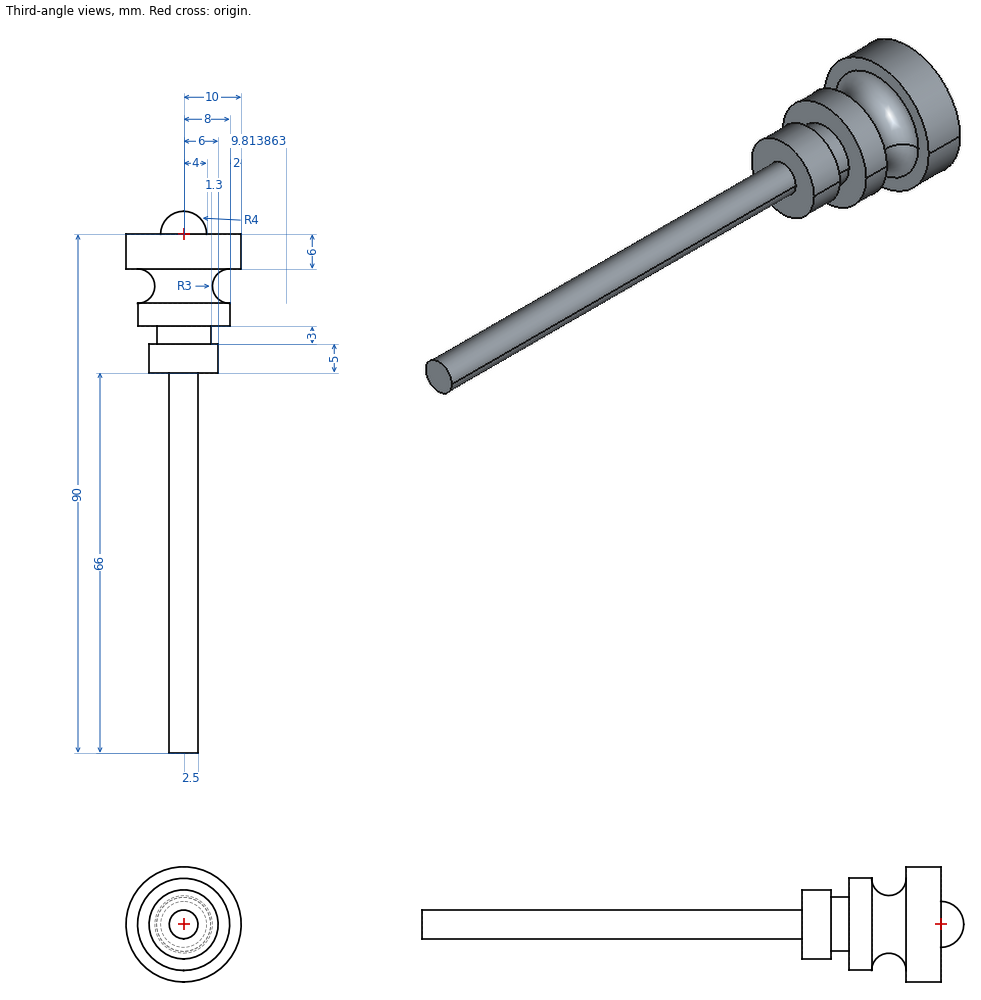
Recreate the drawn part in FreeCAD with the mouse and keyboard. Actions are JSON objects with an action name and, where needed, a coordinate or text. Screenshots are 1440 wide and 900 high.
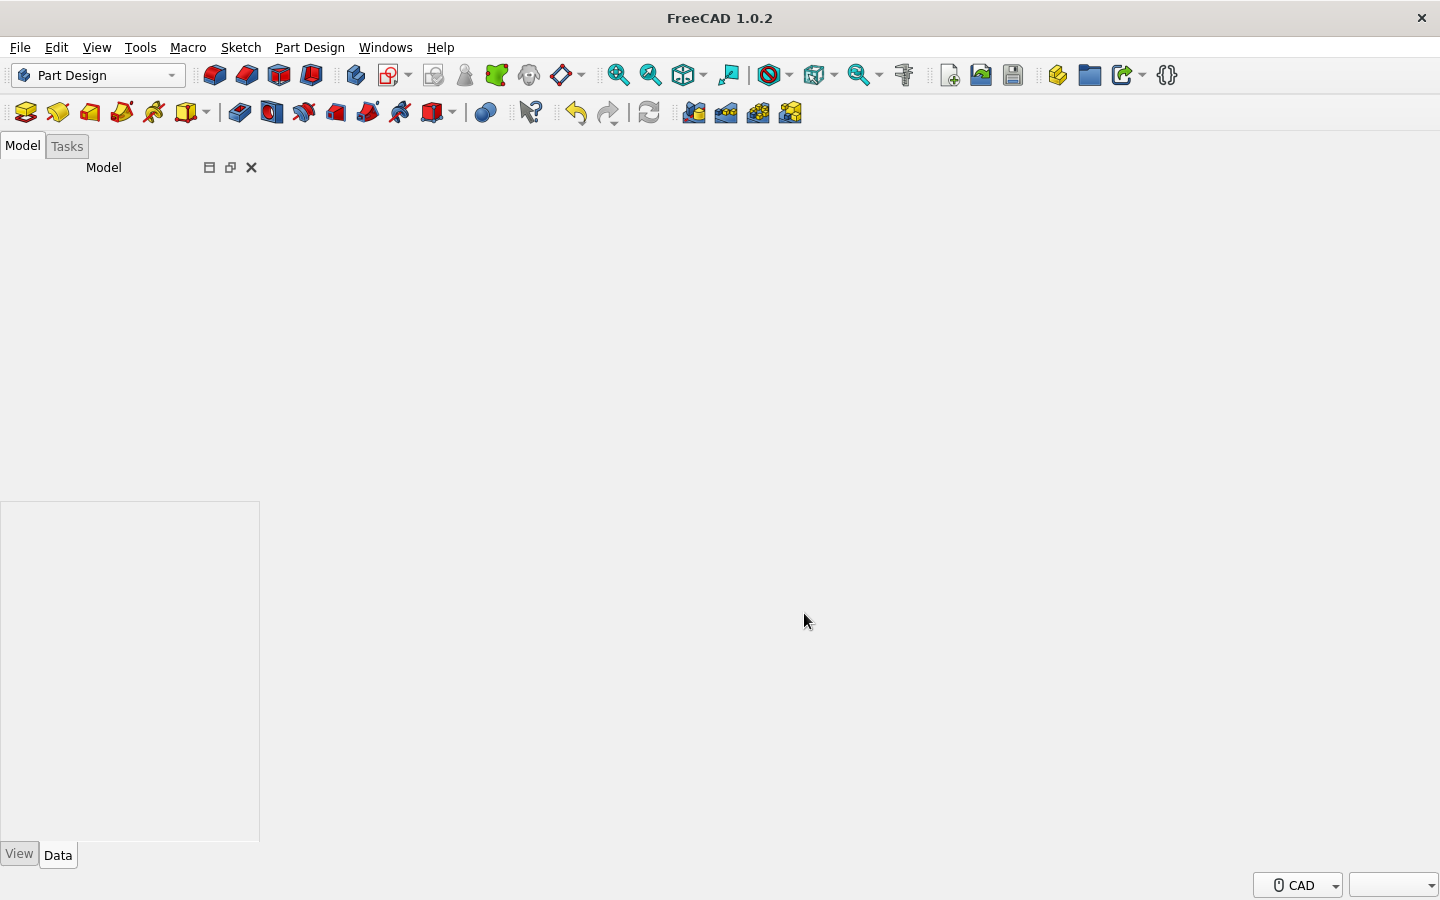
{"action": "key", "text": "ctrl+n"}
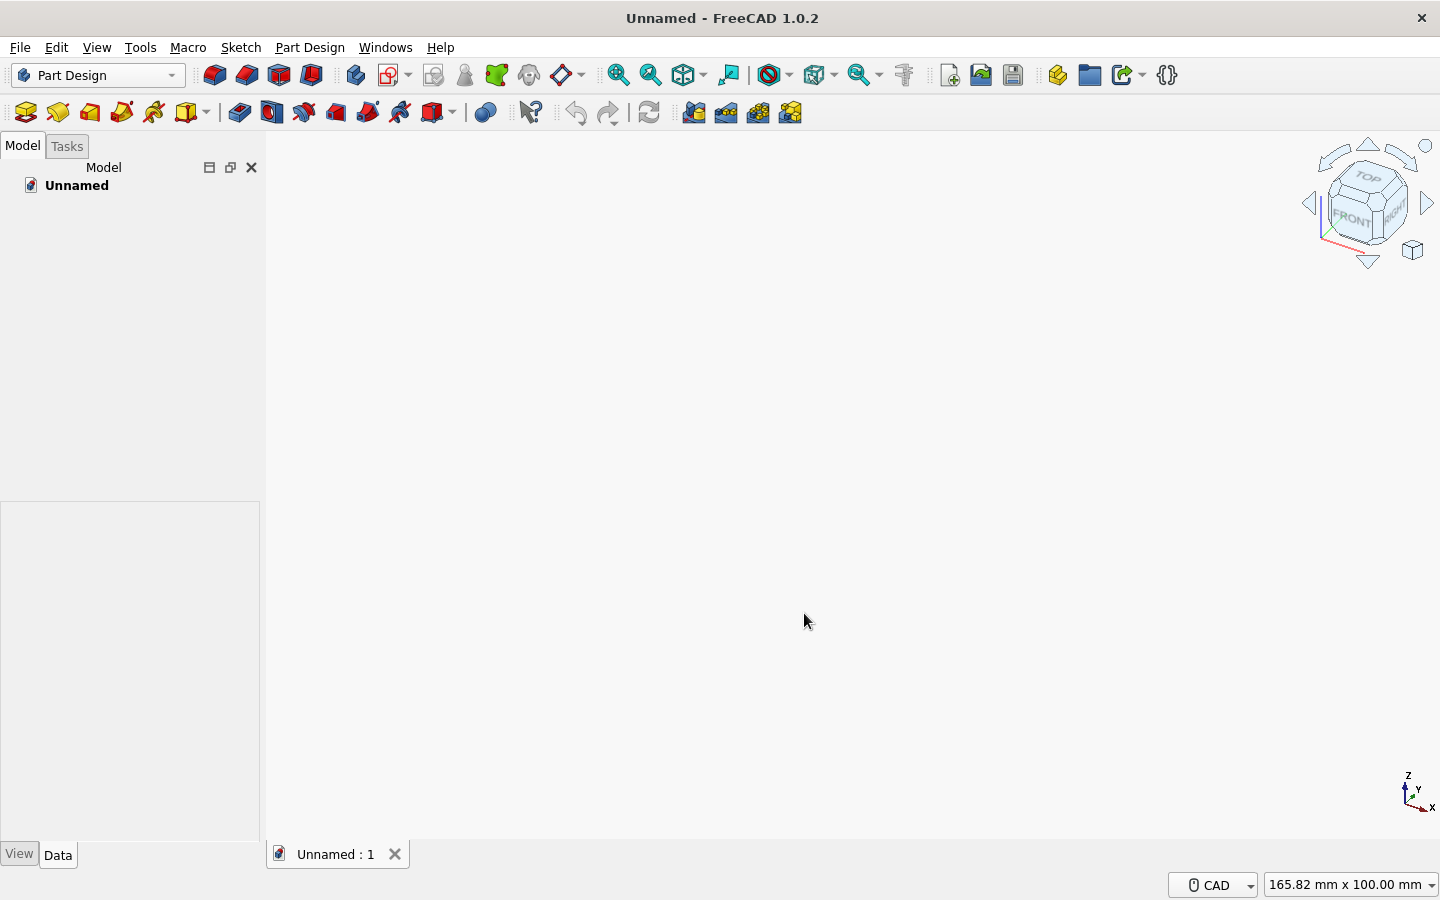
{"action": "left_click", "coordinate": [388, 76]}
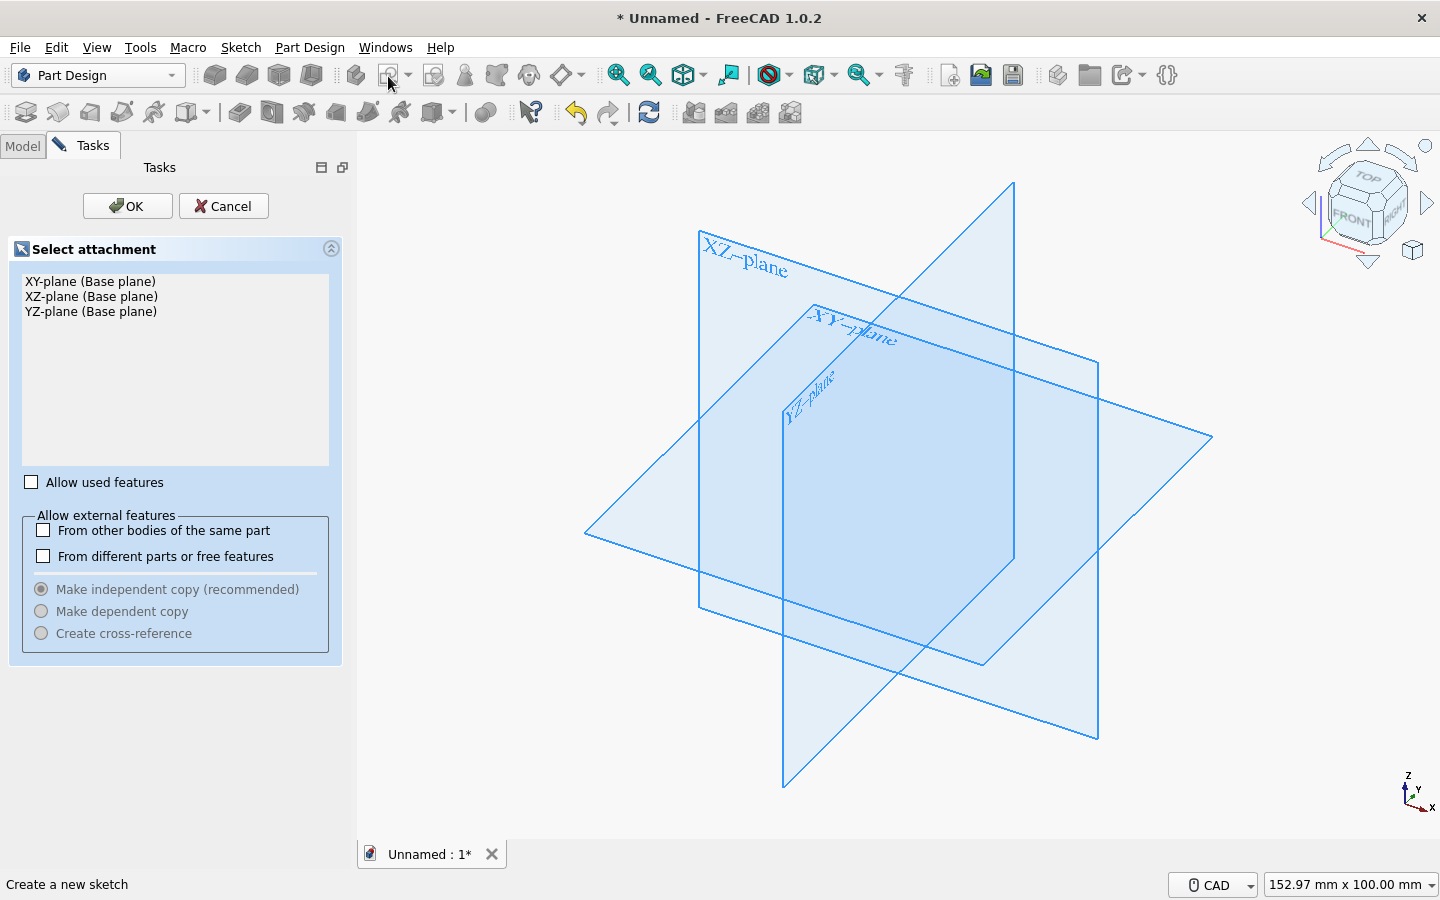
{"action": "left_click", "coordinate": [82, 282]}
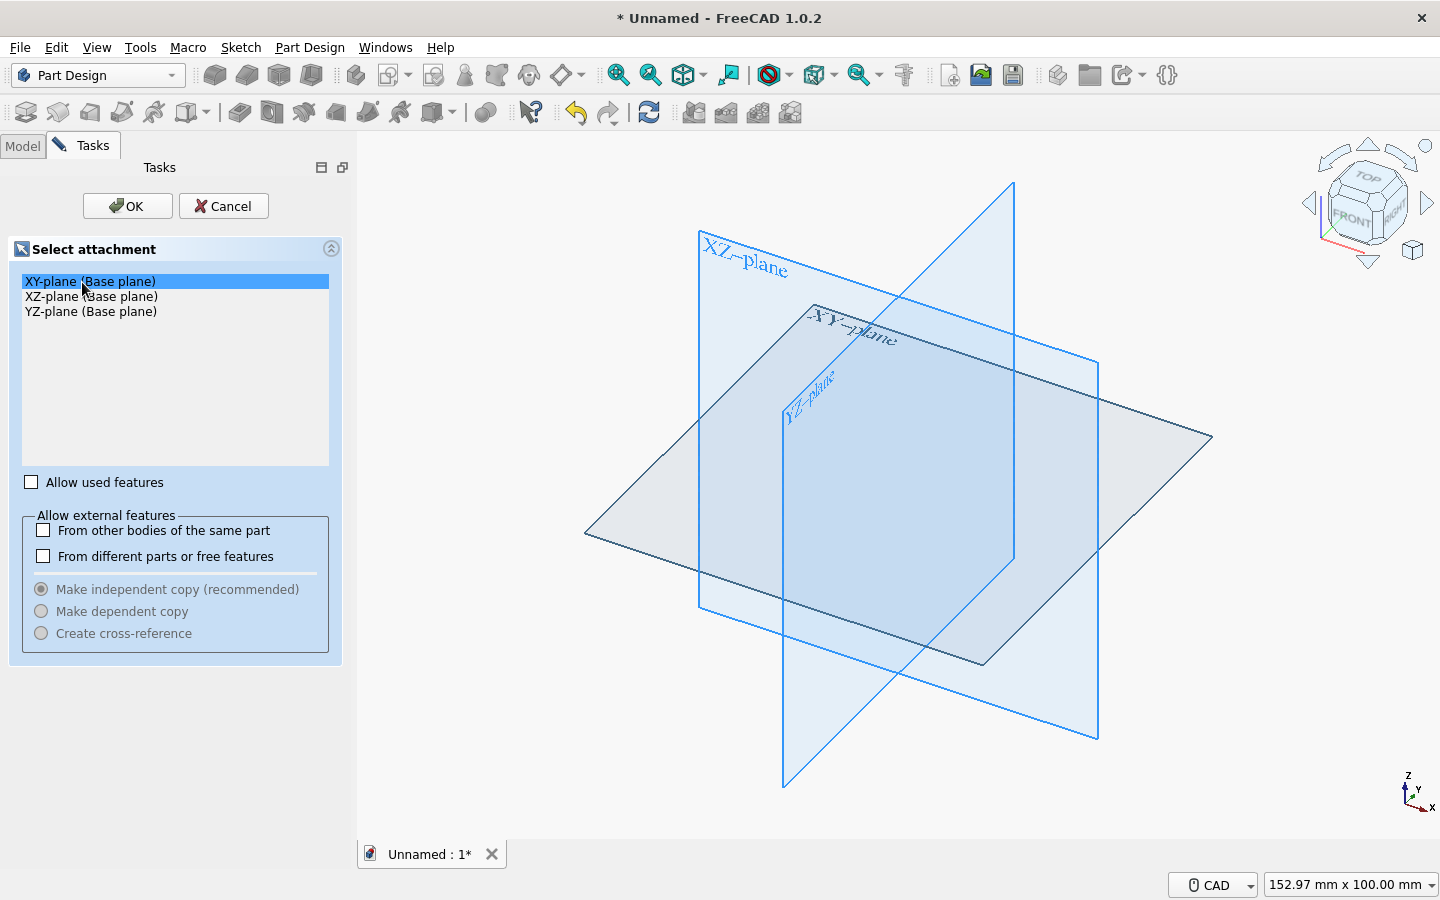
{"action": "left_click", "coordinate": [128, 206]}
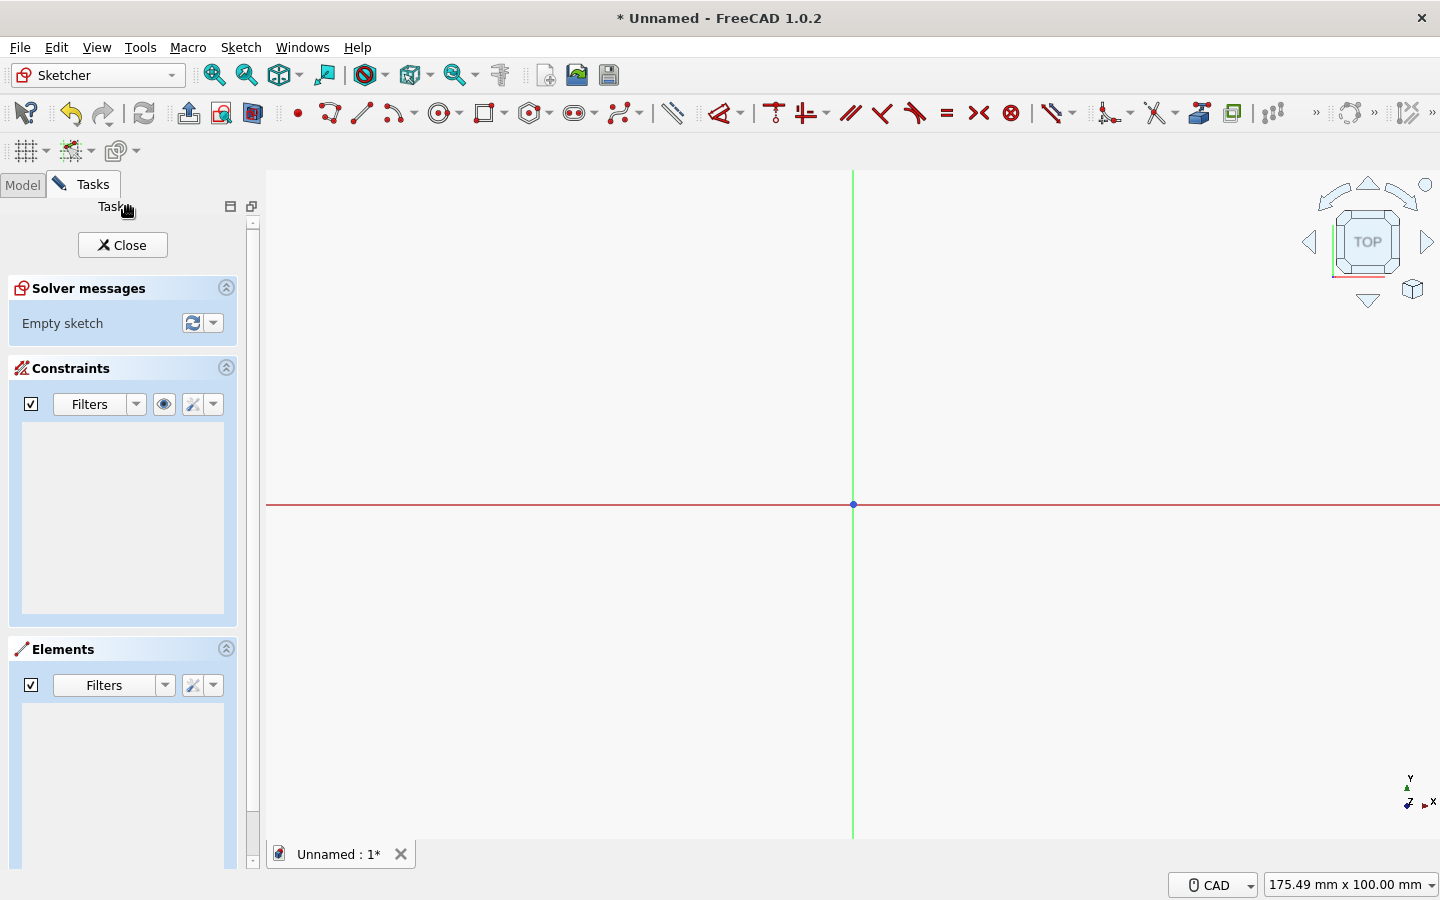
{"action": "scroll", "coordinate": [660, 198], "scroll_direction": "down", "scroll_amount": 3}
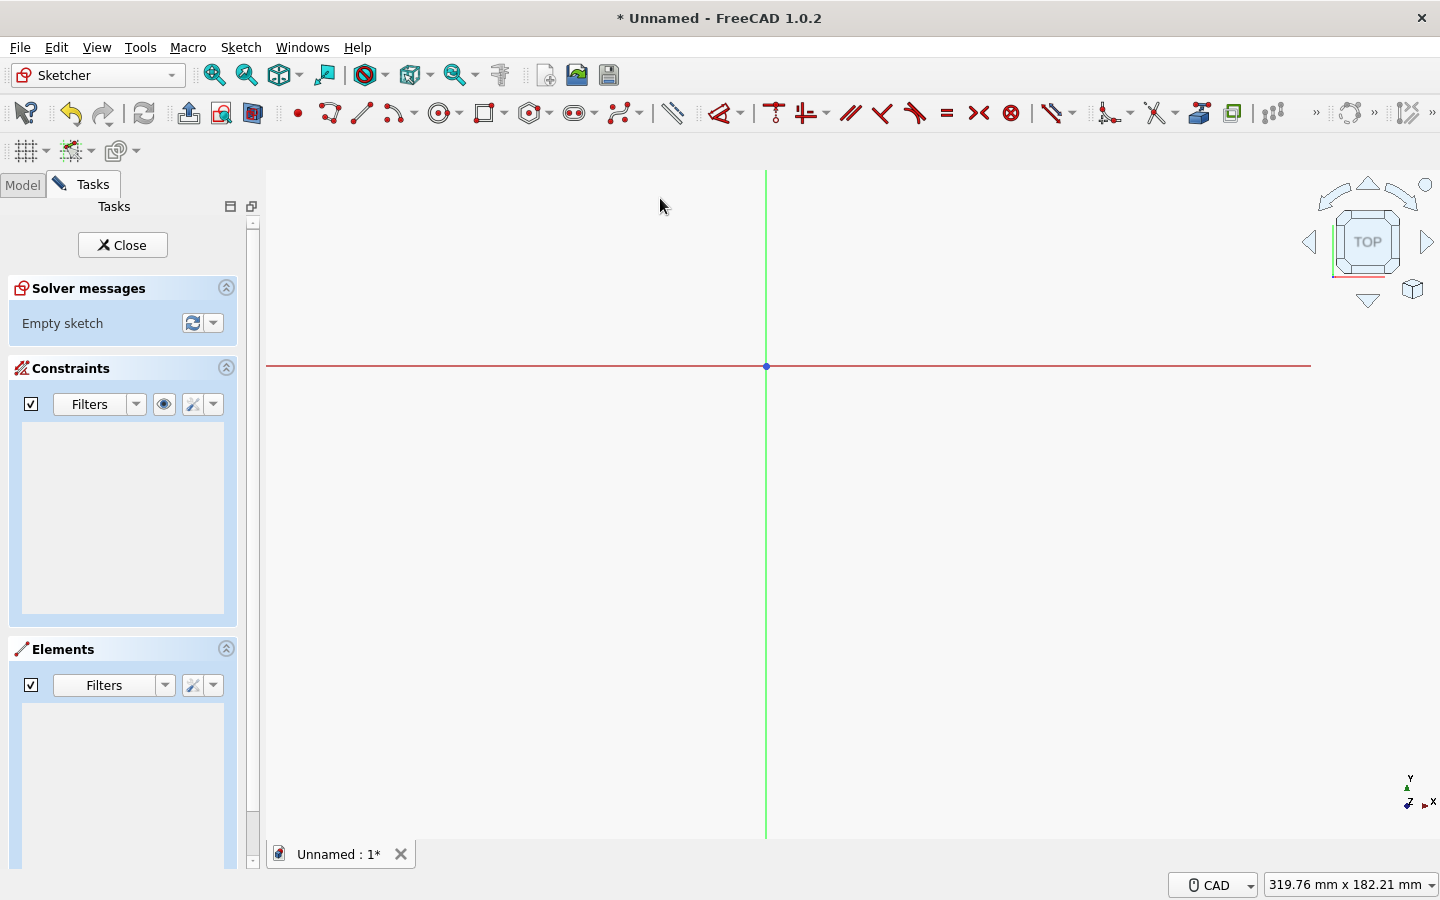
{"action": "key", "text": "g m"}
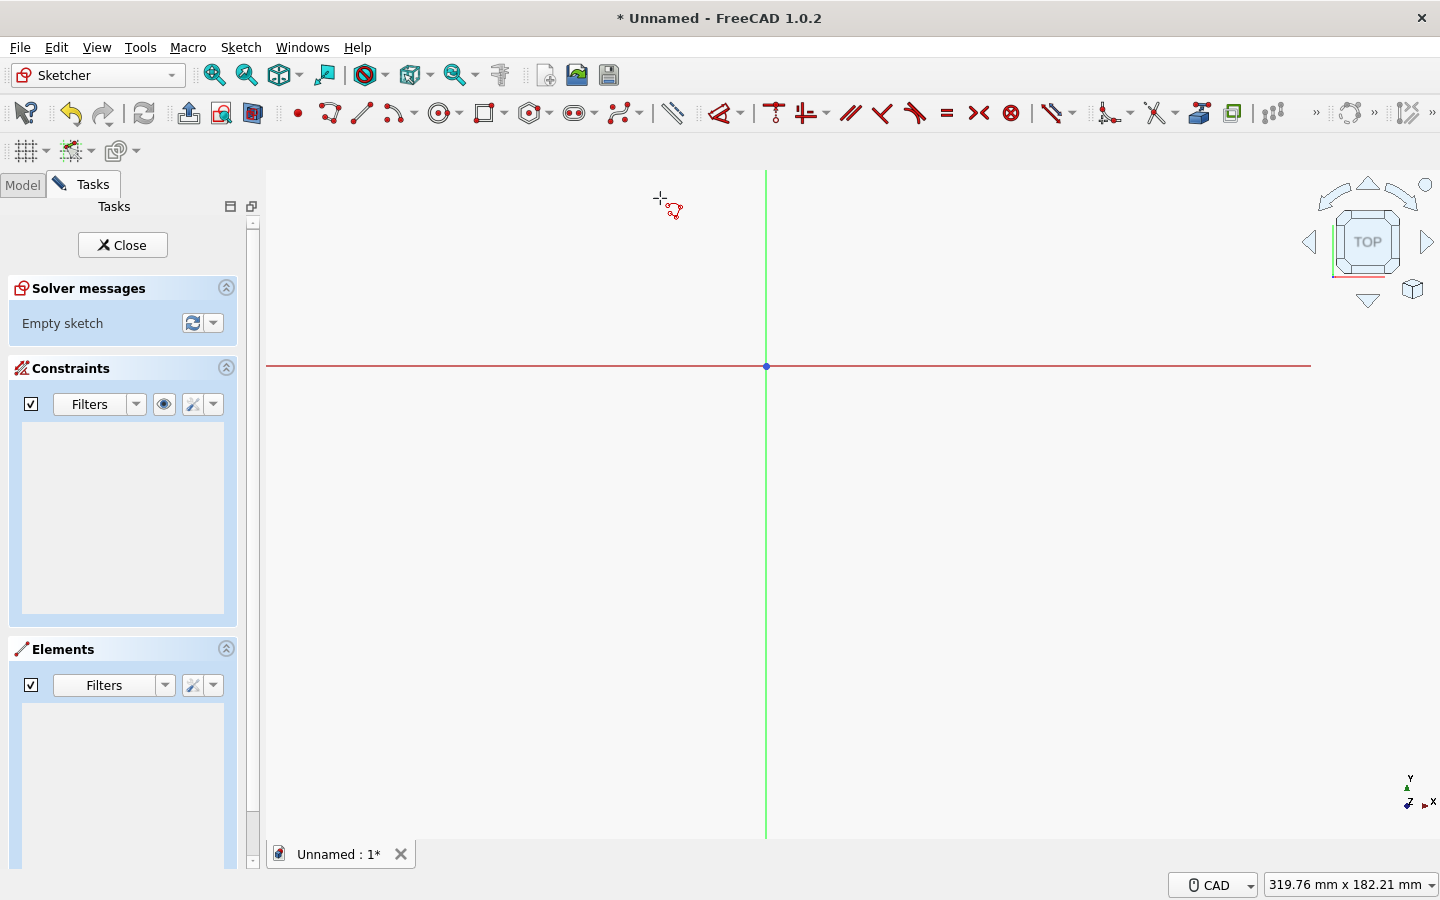
{"action": "left_click", "coordinate": [766, 366]}
{"action": "left_click", "coordinate": [775, 697]}